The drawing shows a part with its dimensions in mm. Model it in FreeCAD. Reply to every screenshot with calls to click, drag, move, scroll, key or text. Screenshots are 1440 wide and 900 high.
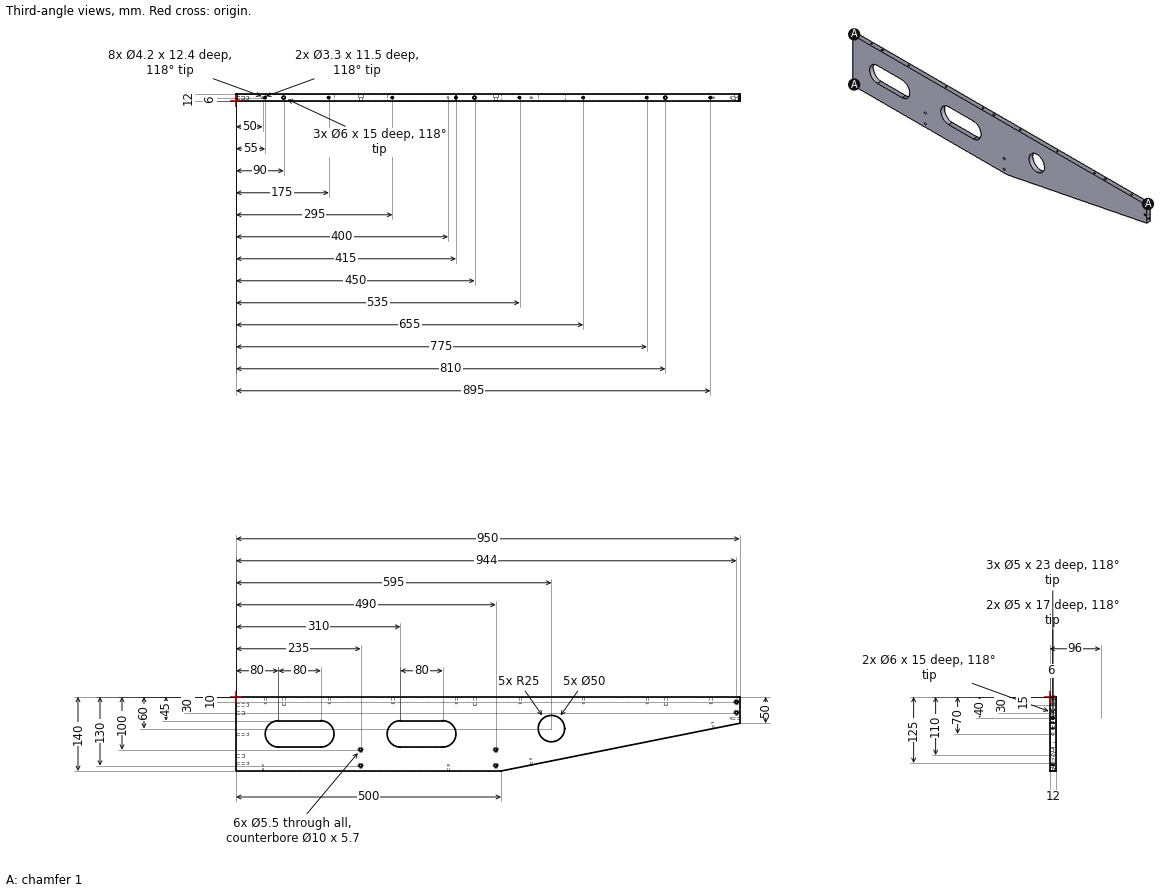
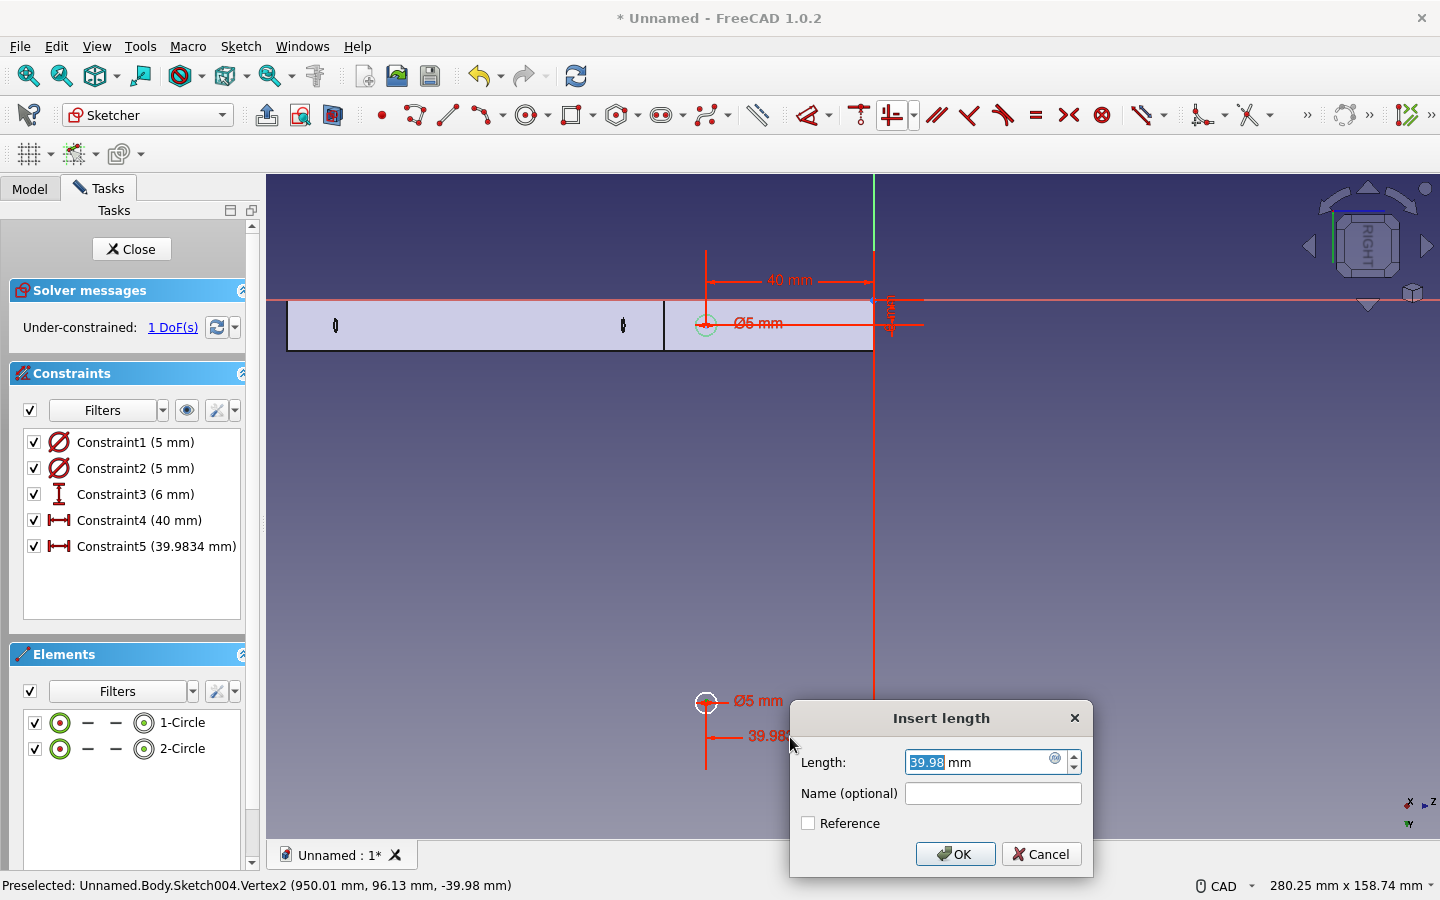
text(40)
key(Return)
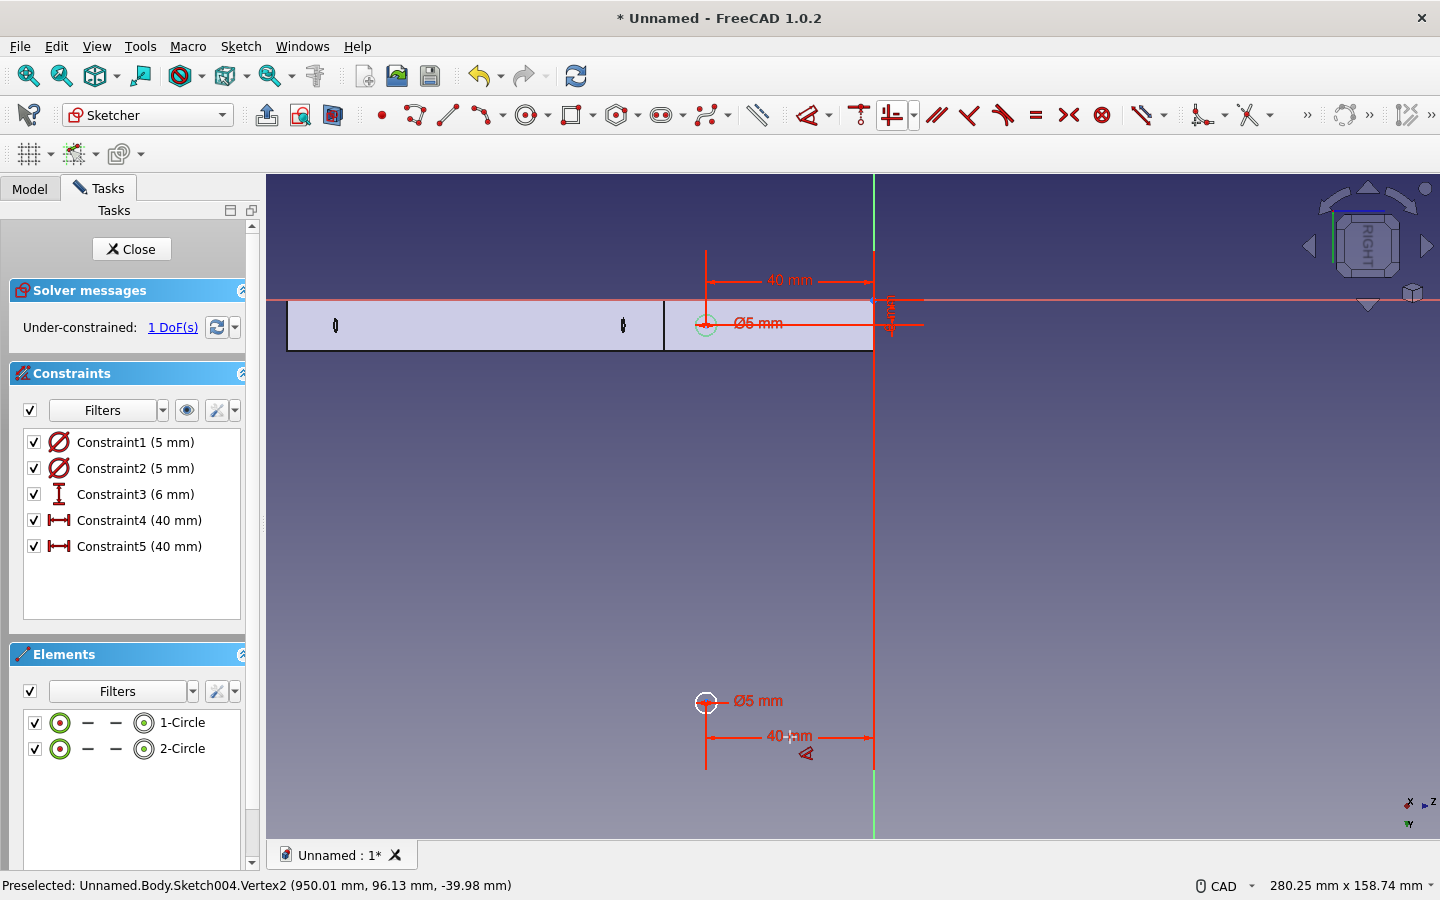
click(706, 703)
click(908, 502)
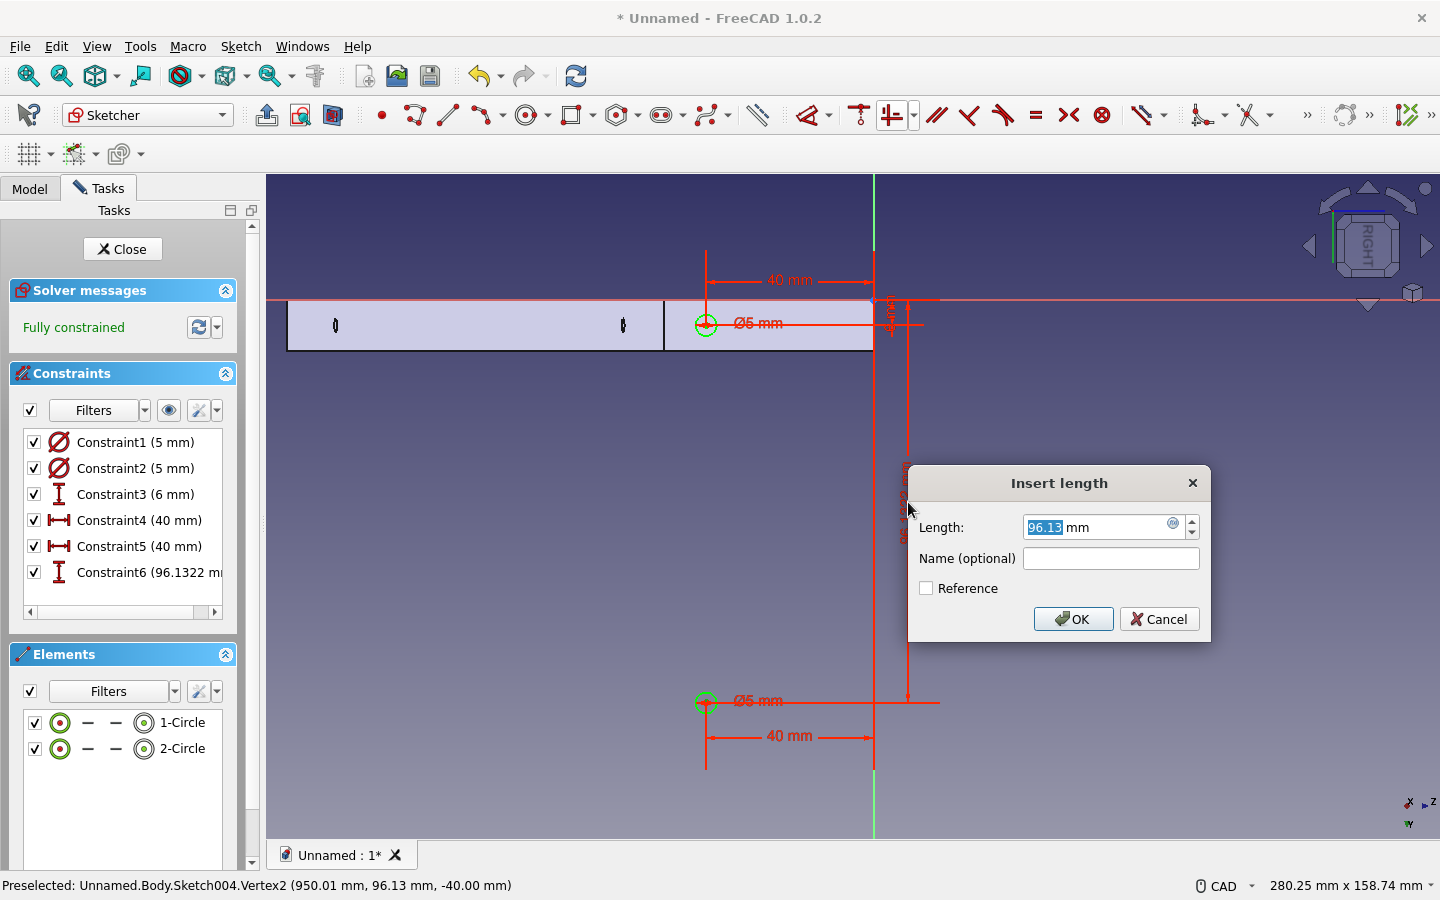
text(96)
key(Return)
key(Escape)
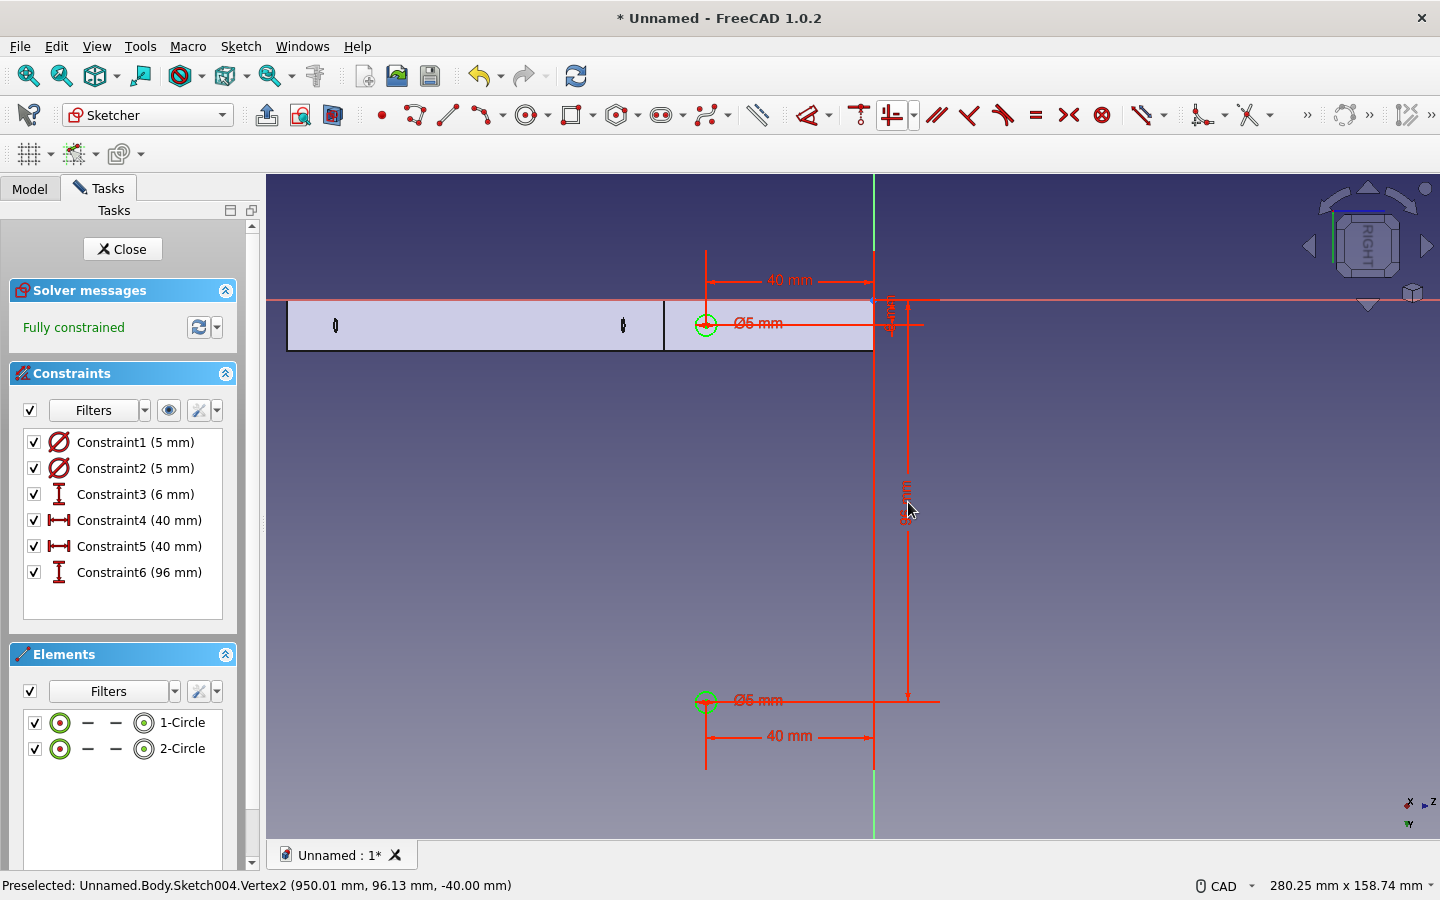
click(123, 249)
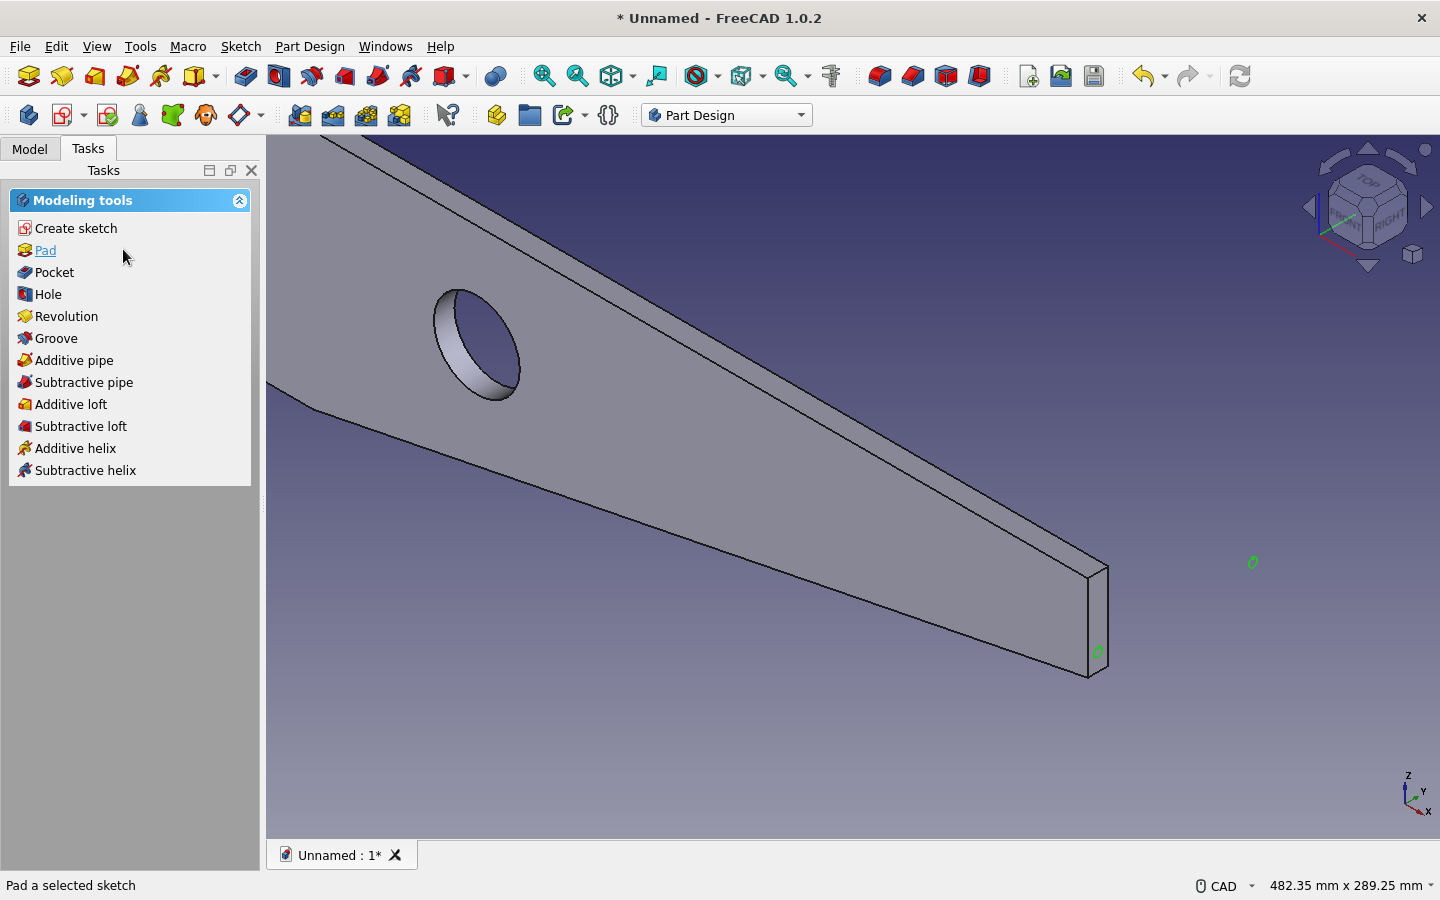
click(279, 76)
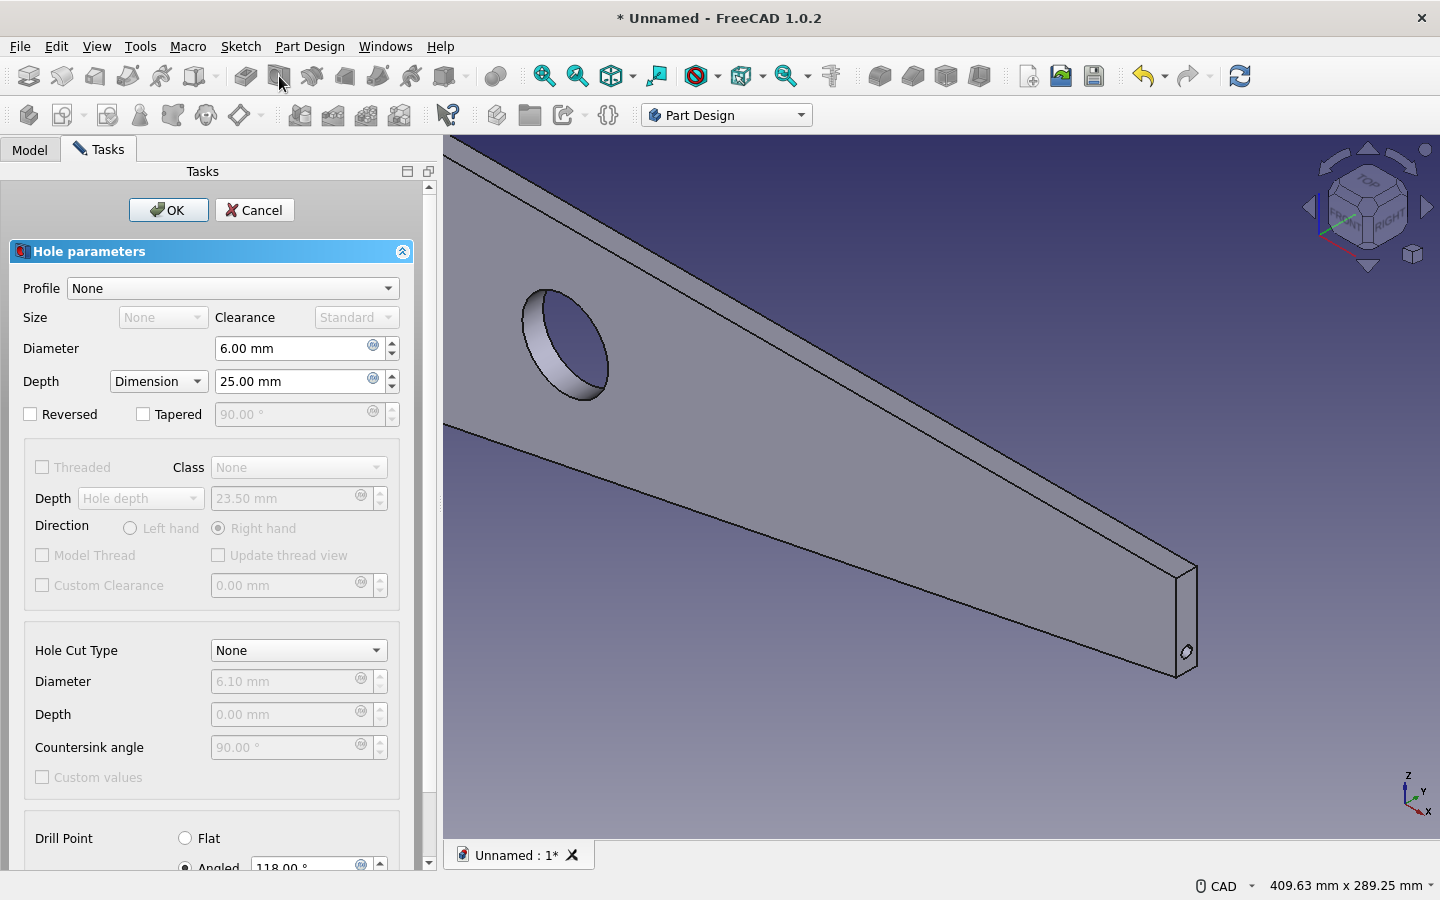
triple_click(300, 348)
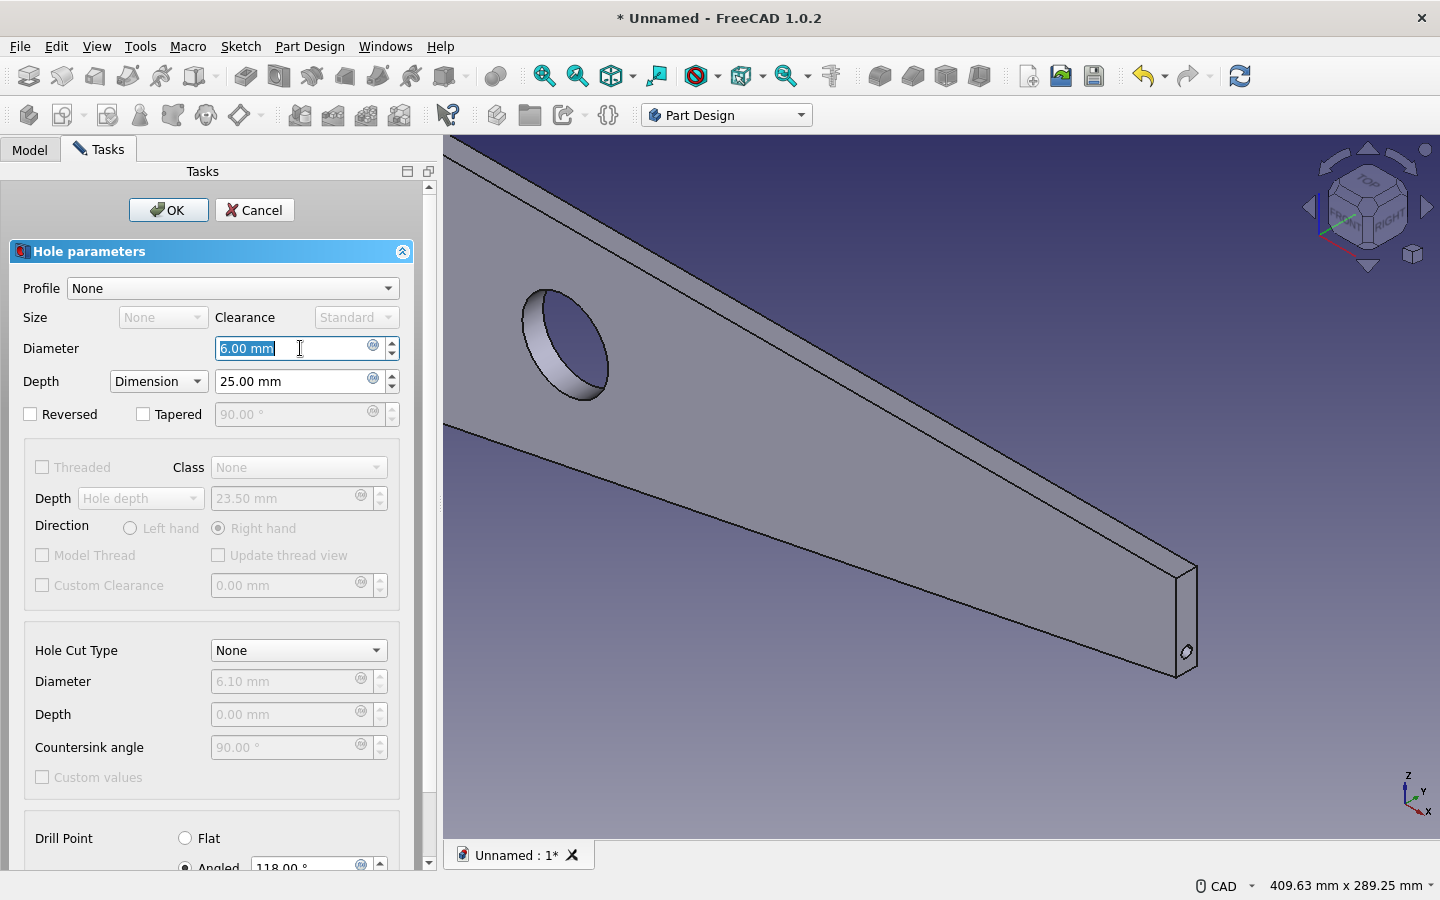
text(5)
key(Tab)